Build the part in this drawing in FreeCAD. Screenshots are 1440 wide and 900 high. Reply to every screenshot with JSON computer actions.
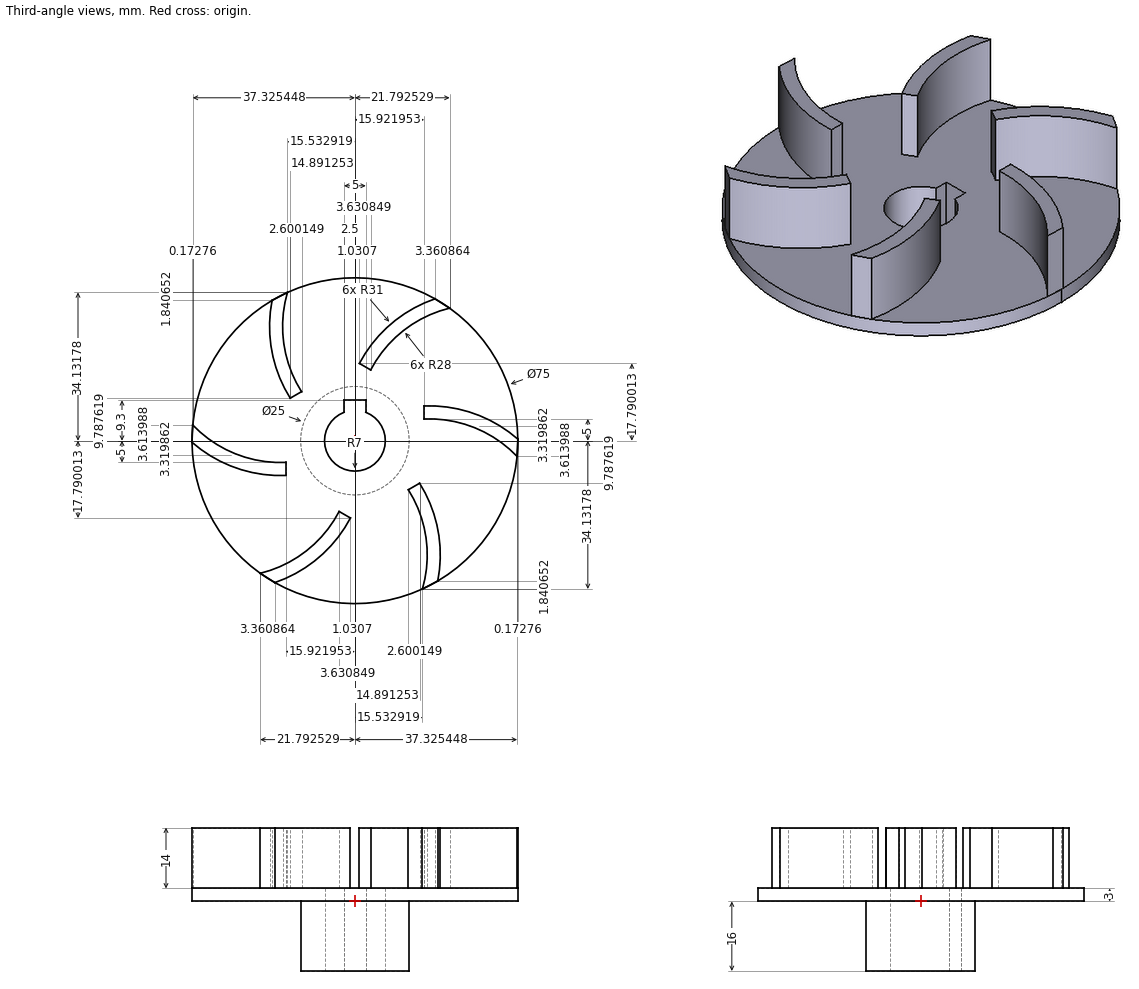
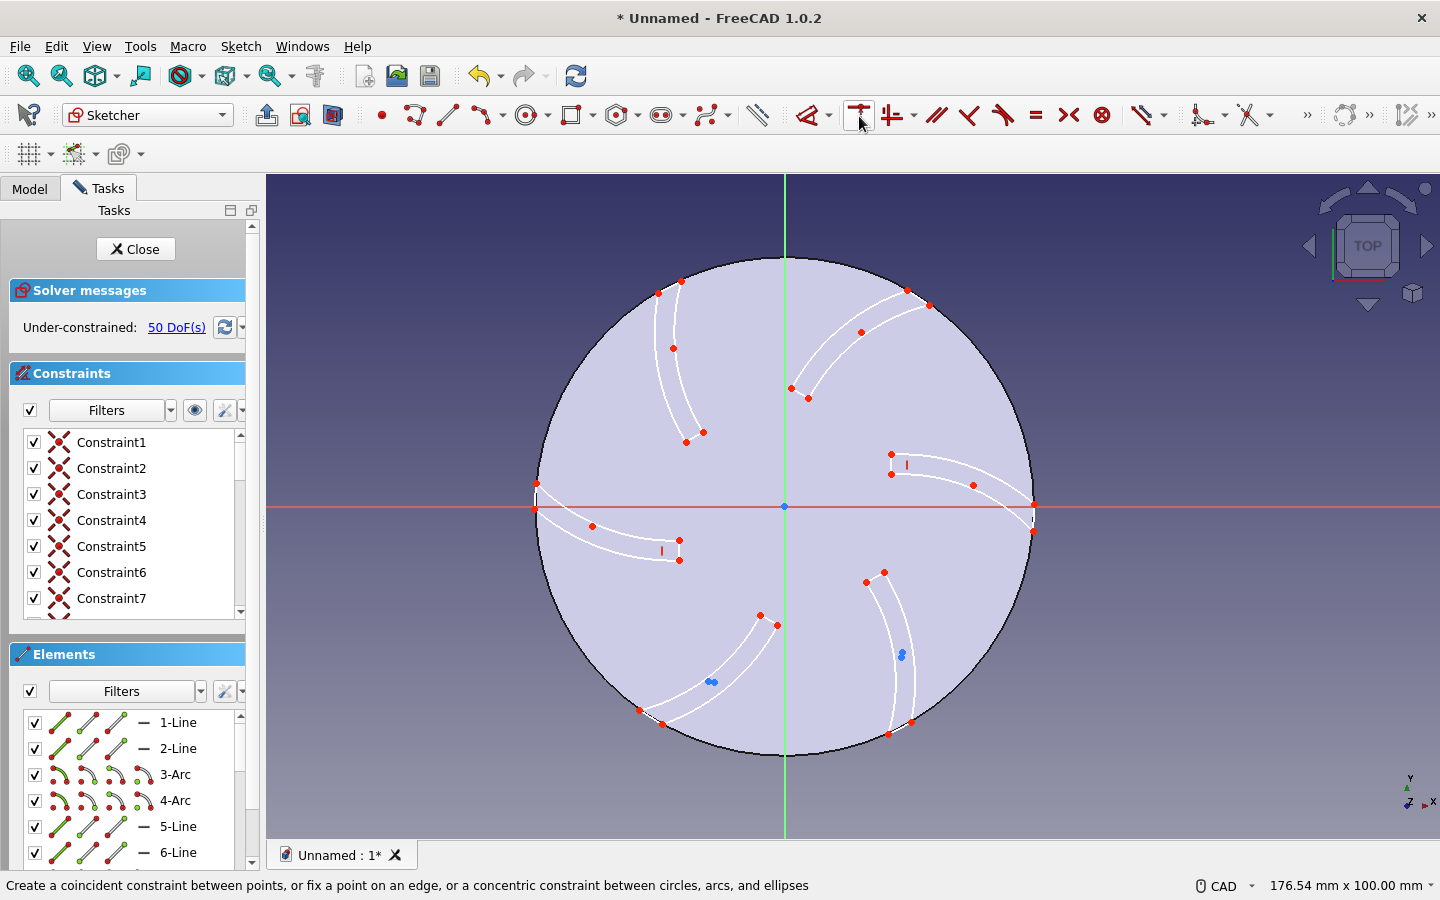
{"action": "left_click", "coordinate": [915, 676]}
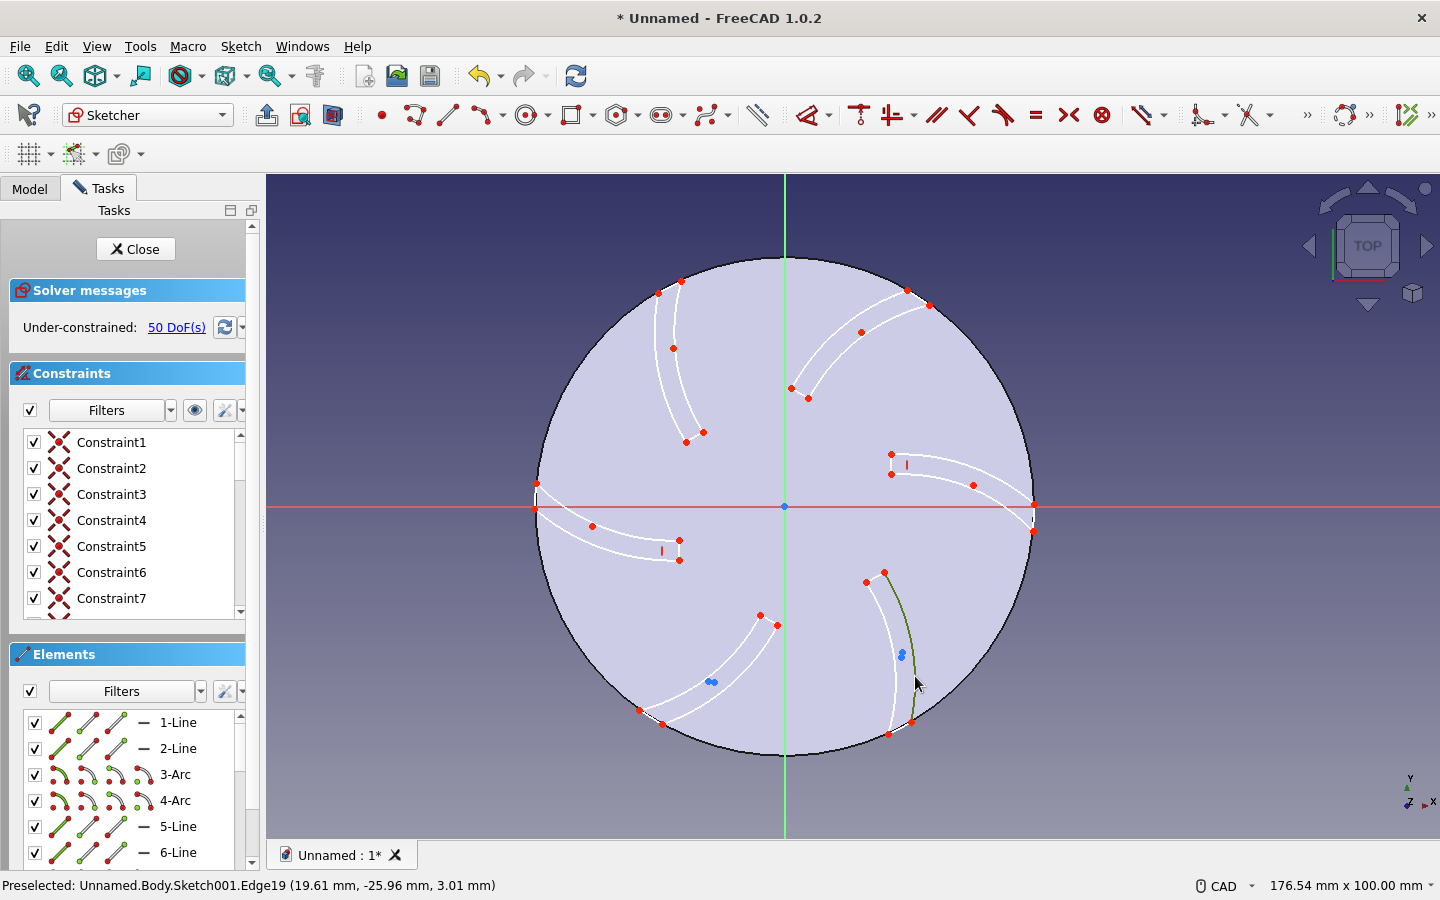
{"action": "left_click", "coordinate": [896, 688]}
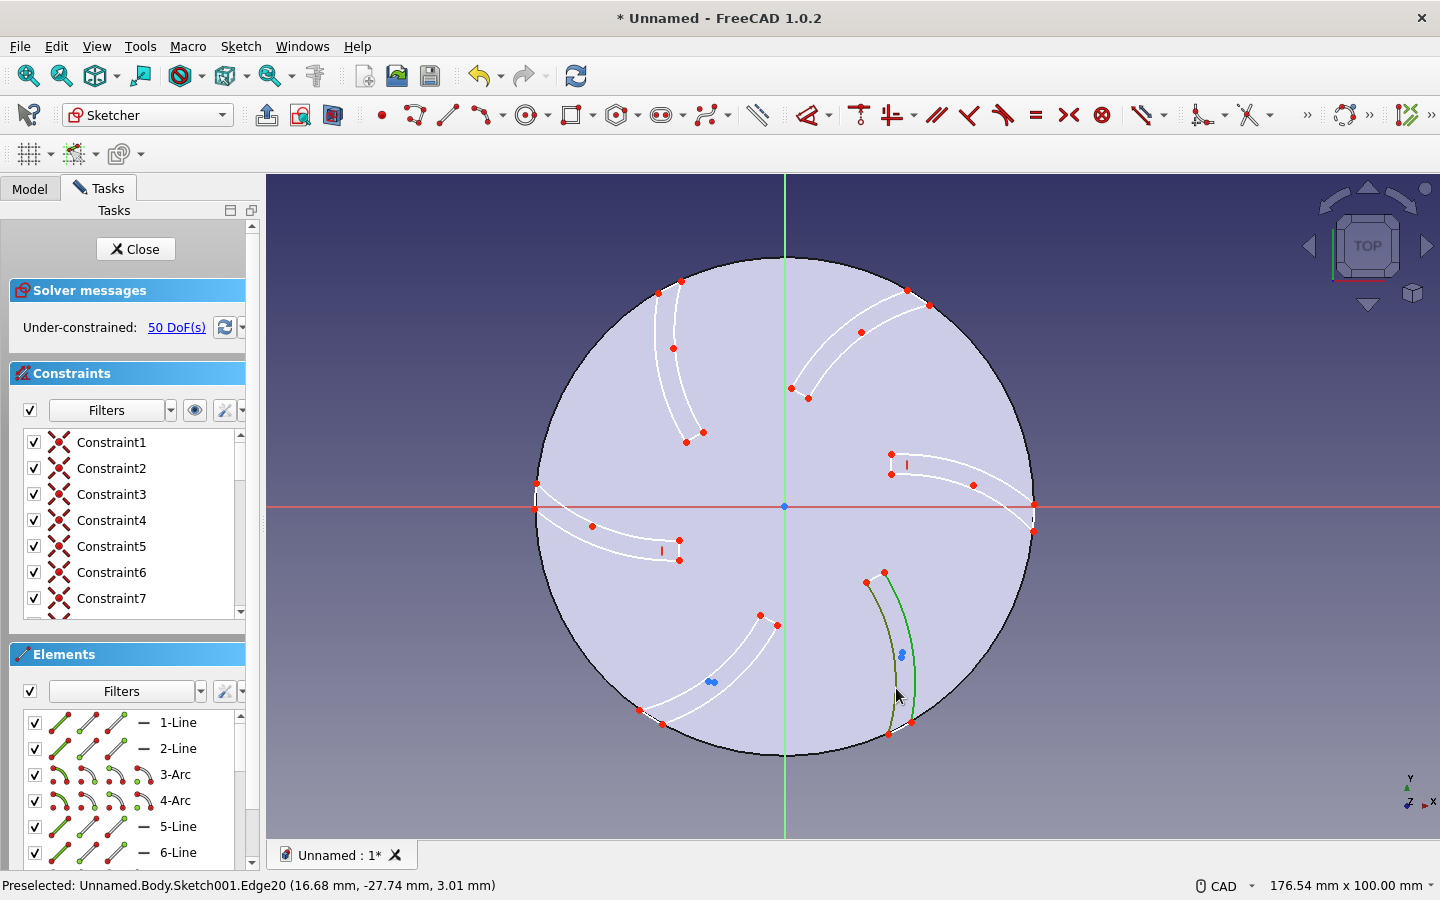
{"action": "key", "text": "c"}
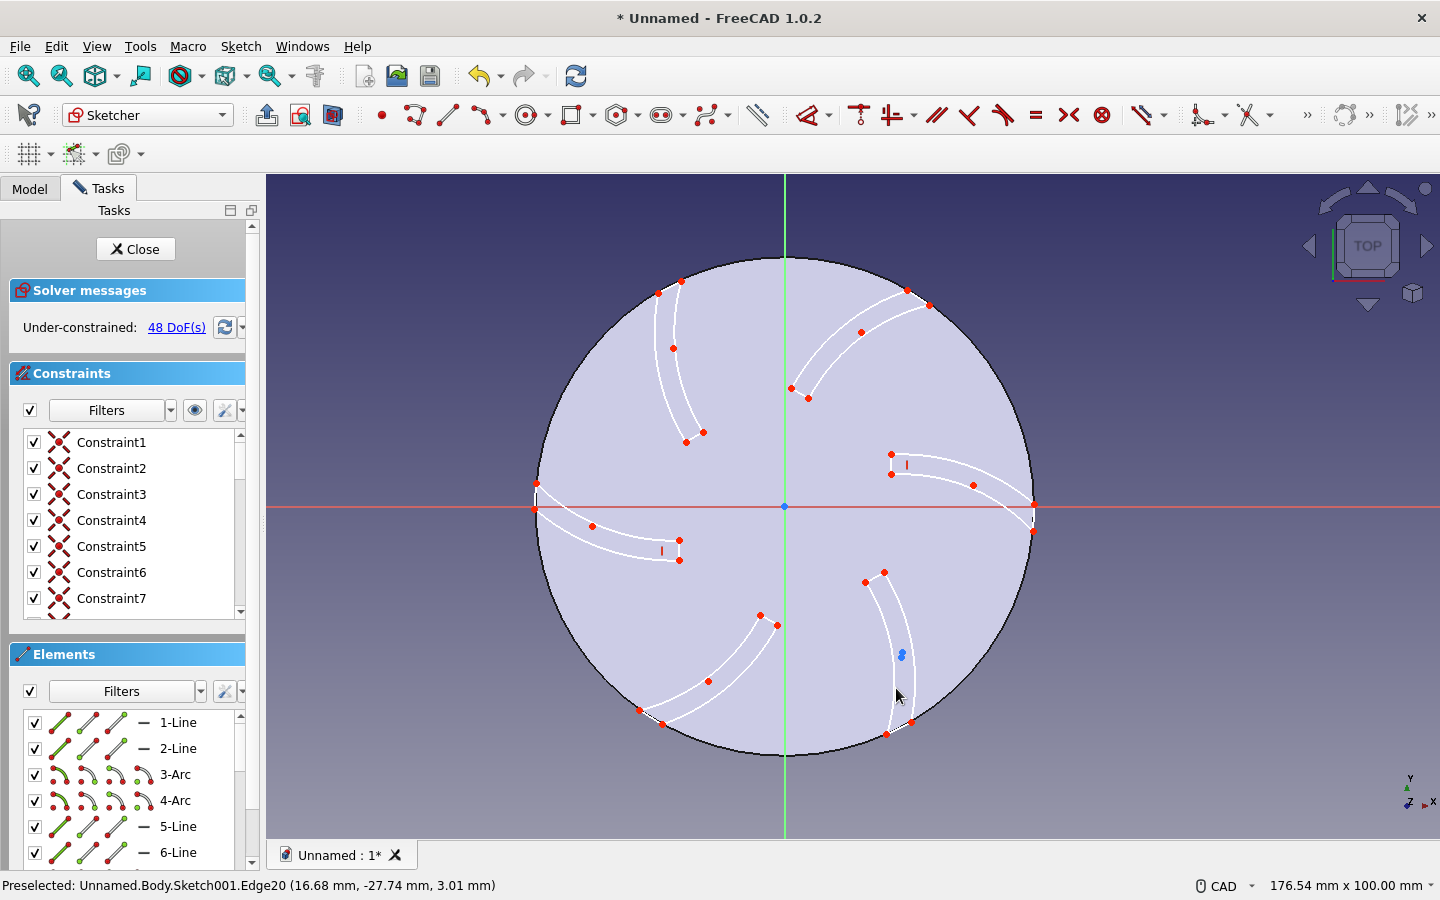
{"action": "left_click", "coordinate": [996, 478]}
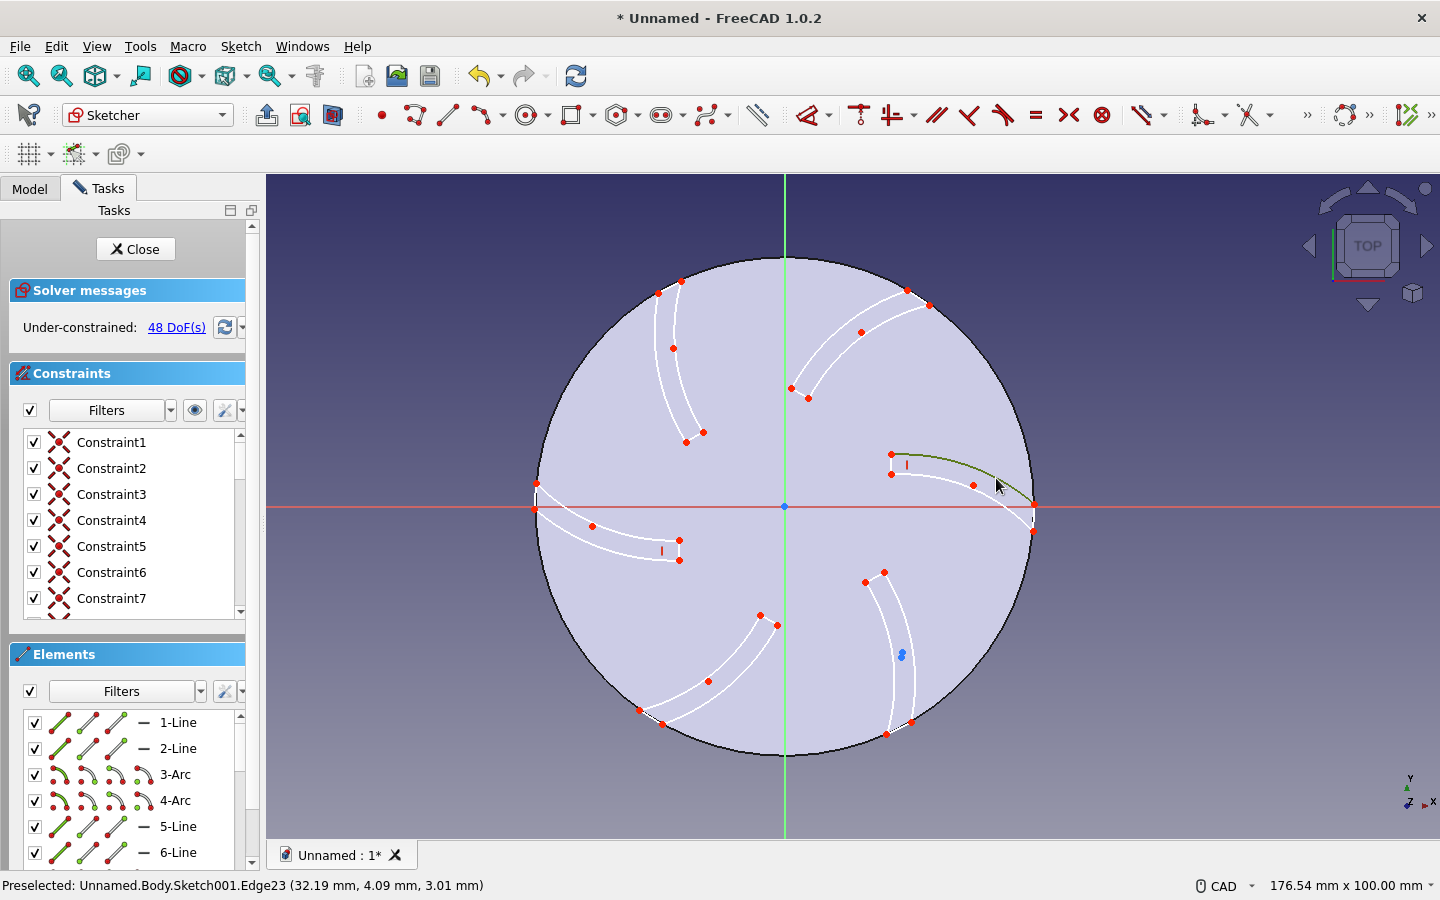
{"action": "left_click", "coordinate": [938, 478]}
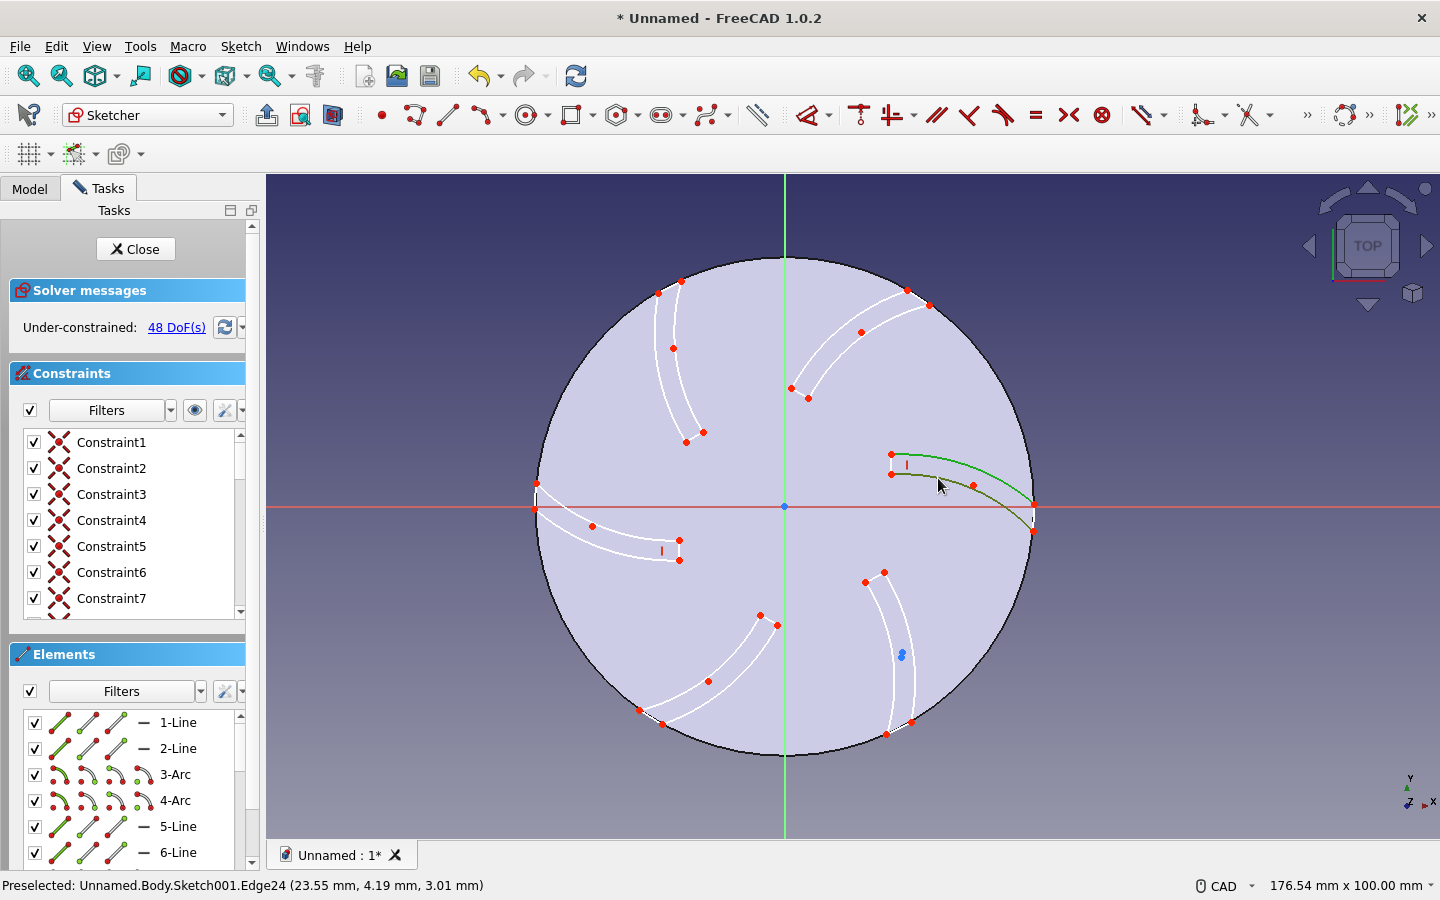
{"action": "left_click", "coordinate": [859, 116]}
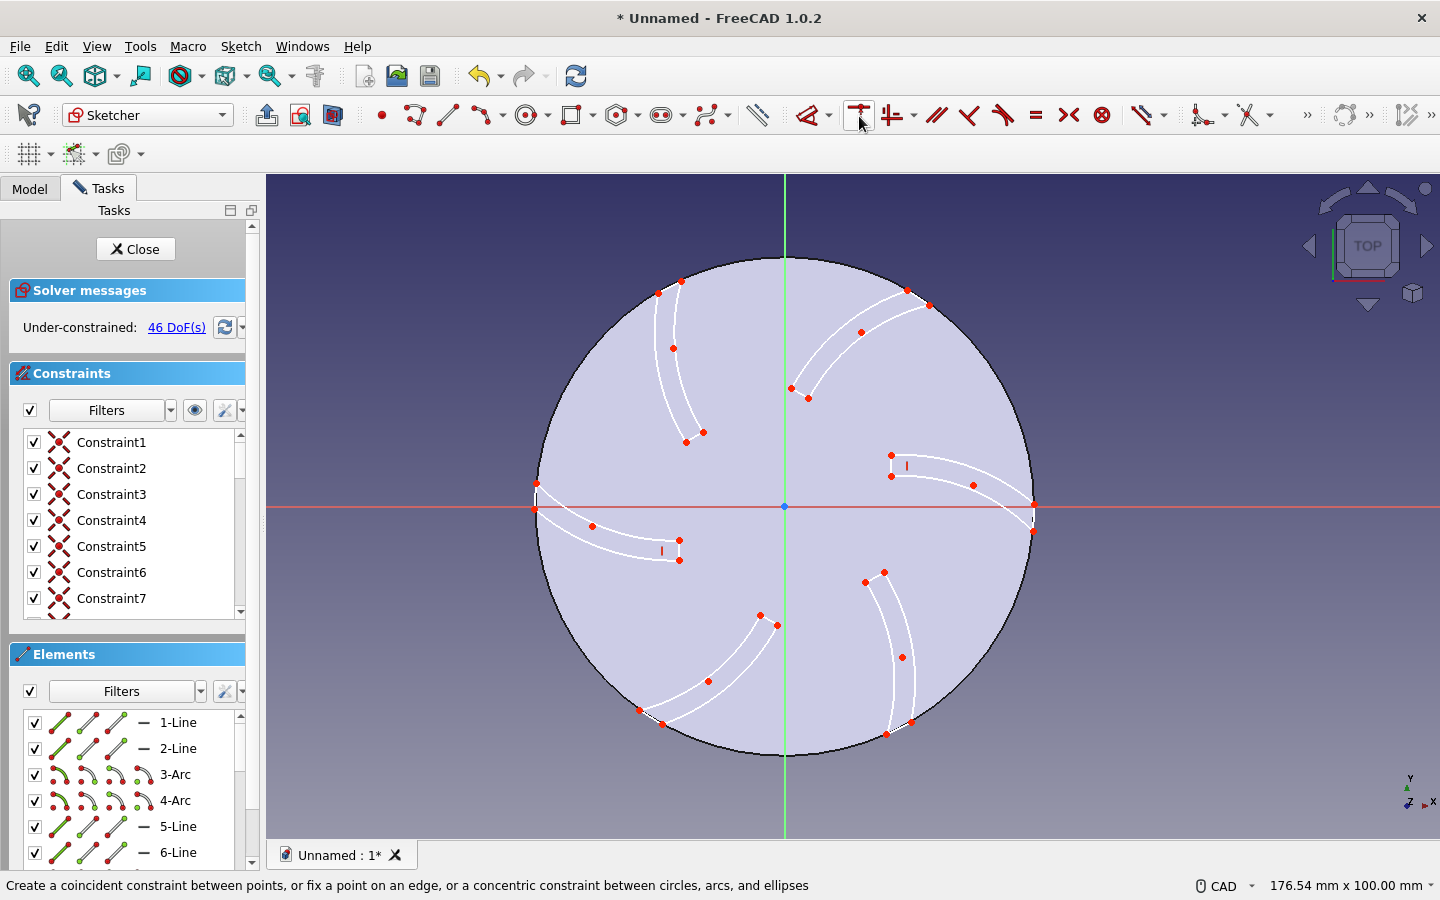
{"action": "left_click", "coordinate": [865, 310]}